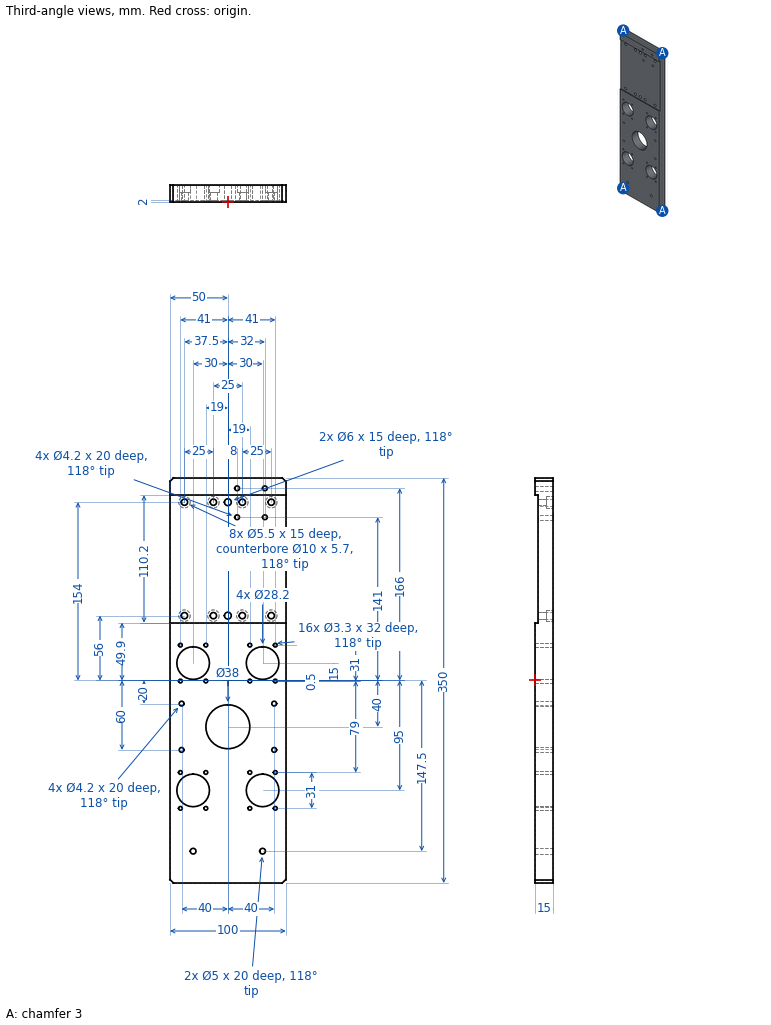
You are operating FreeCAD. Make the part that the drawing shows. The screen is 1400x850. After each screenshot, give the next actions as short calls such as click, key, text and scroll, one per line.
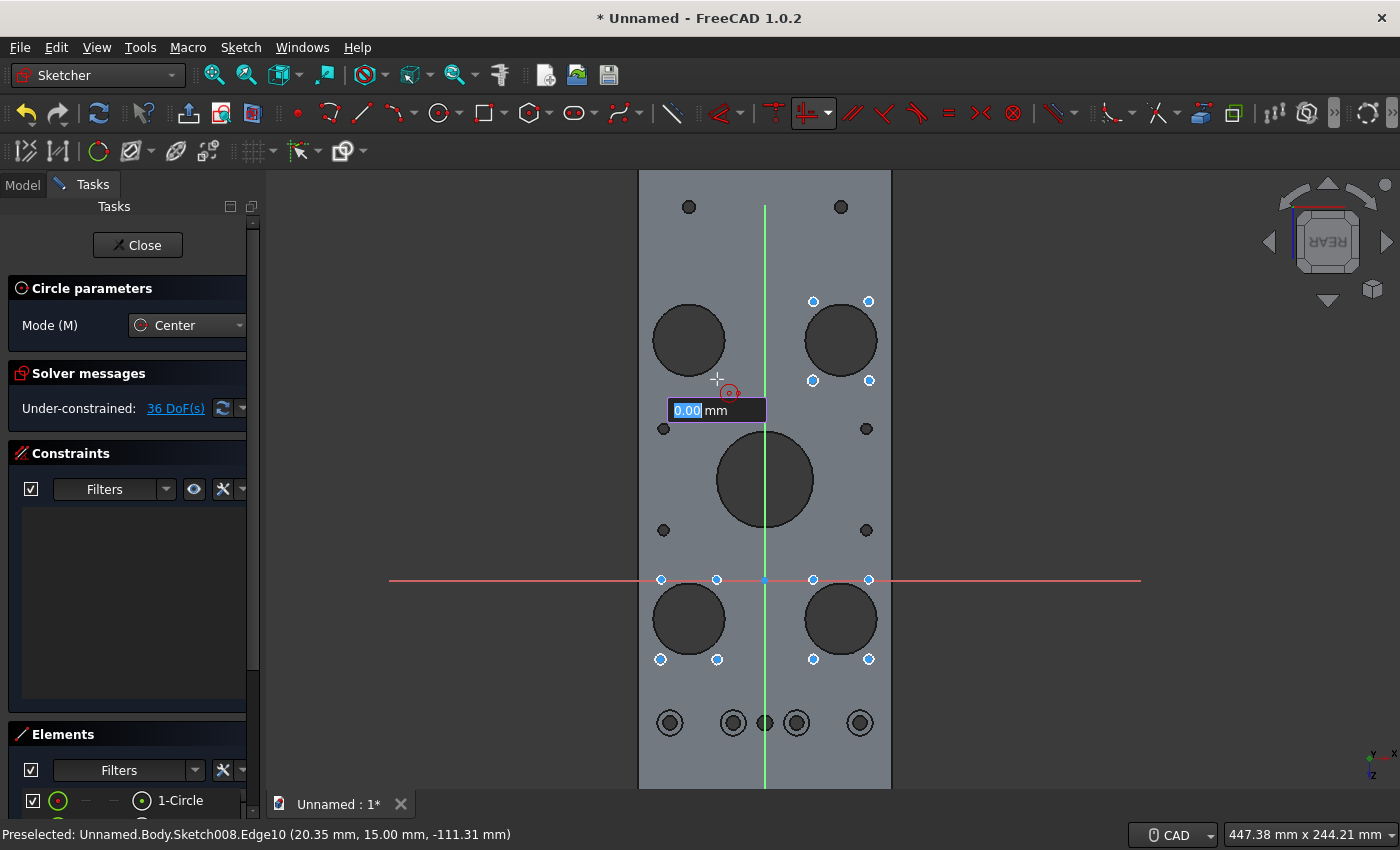
scroll(720, 377, up, 7)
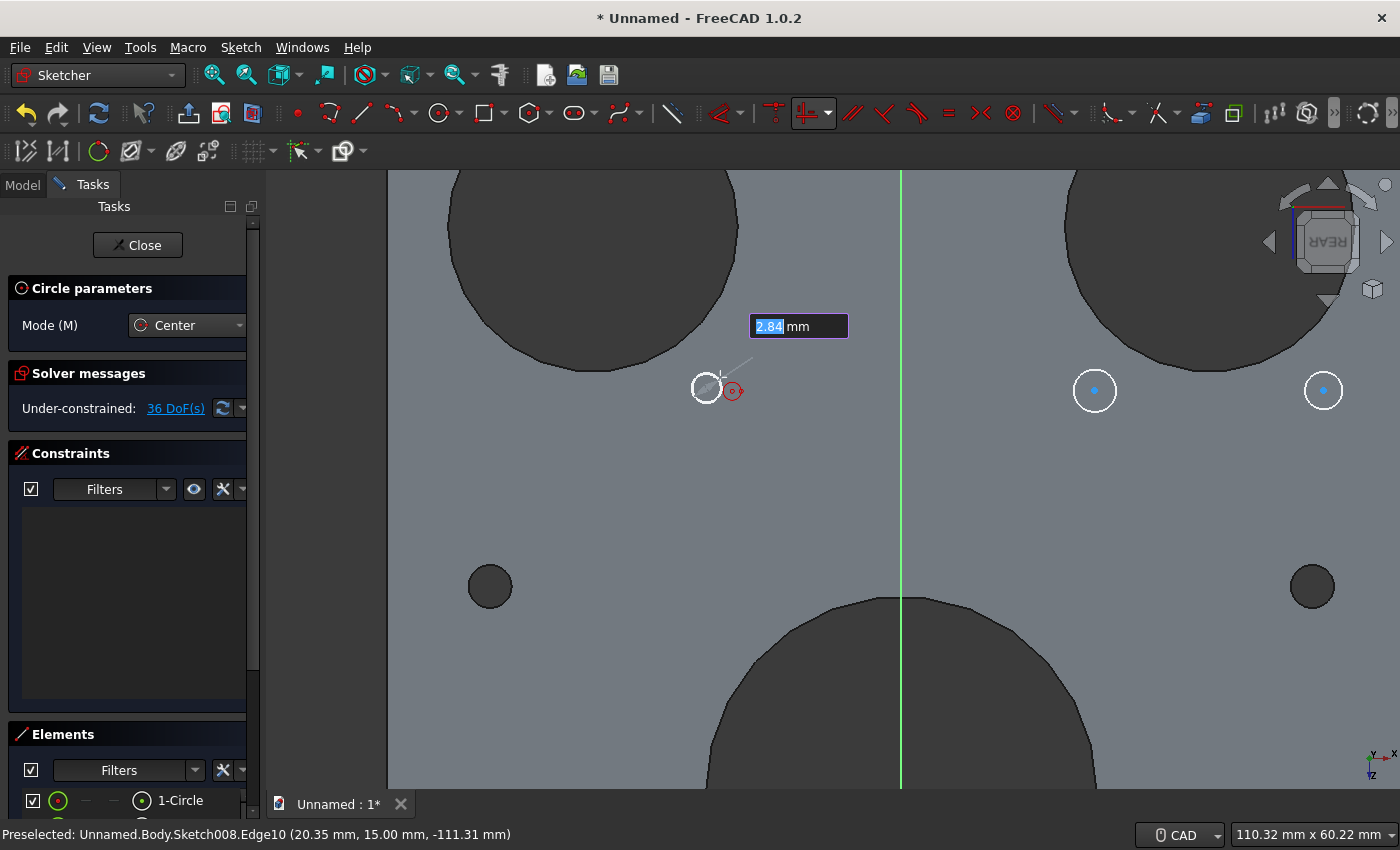
click(718, 374)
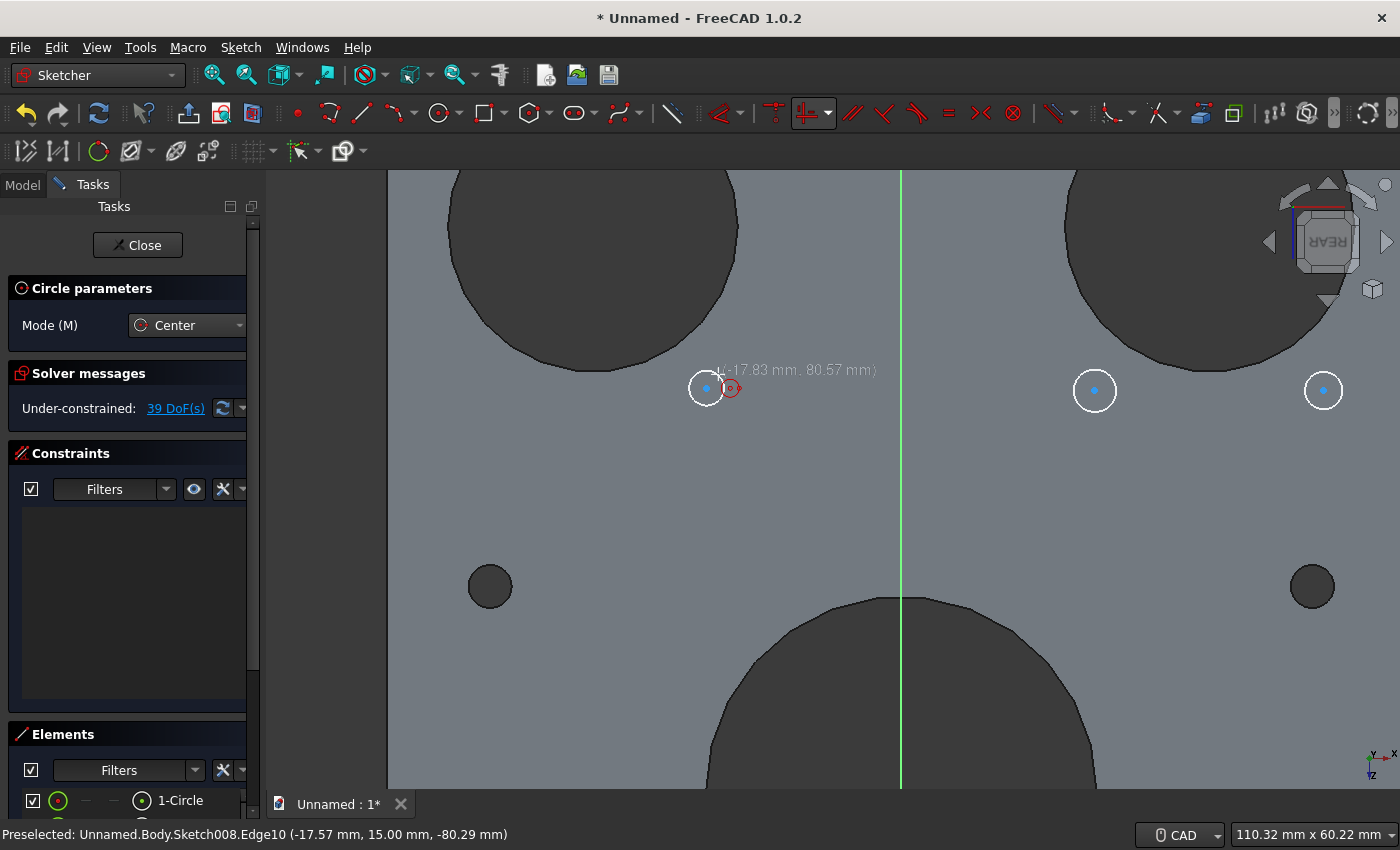
scroll(480, 386, up, 2)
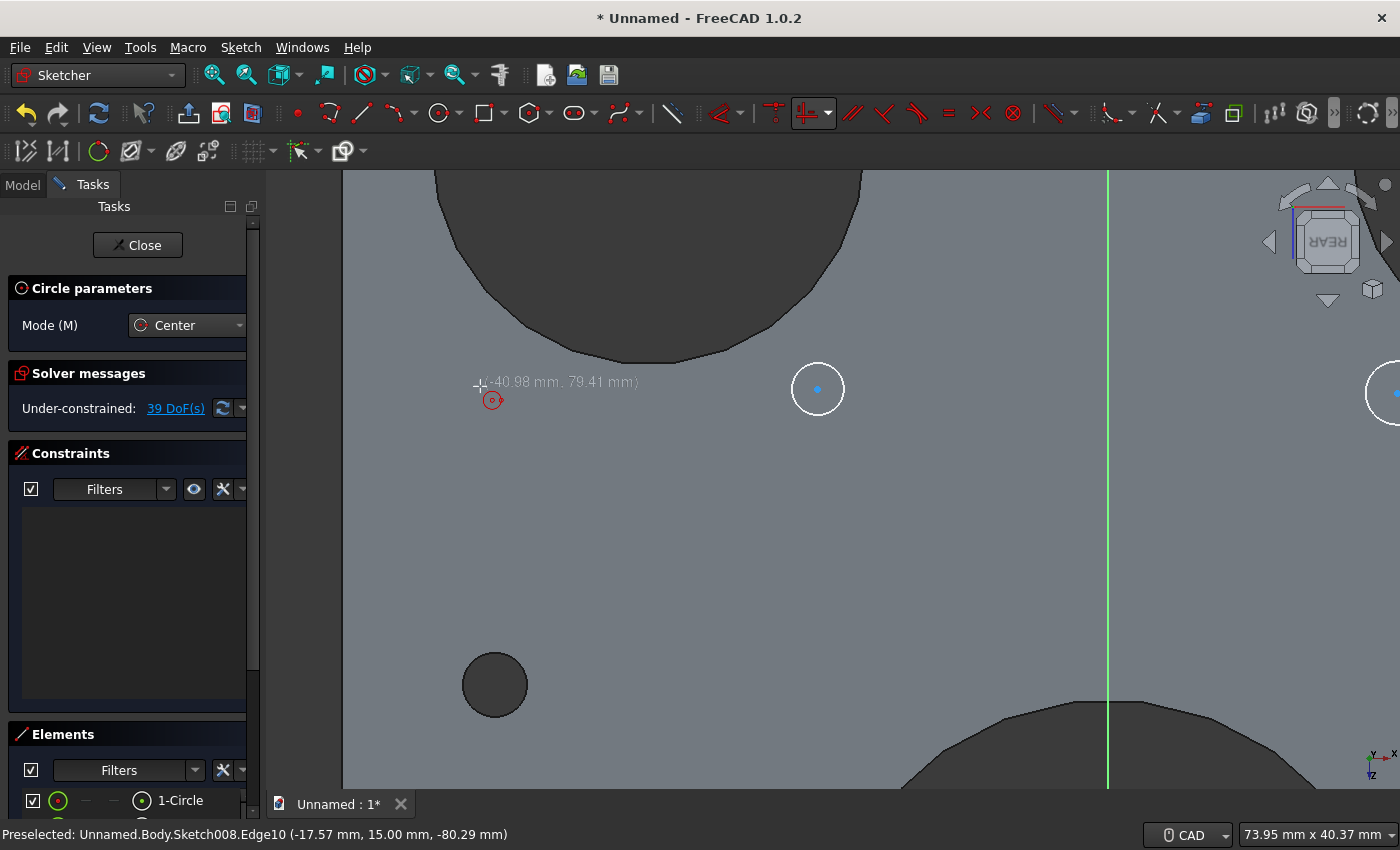
scroll(696, 378, down, 9)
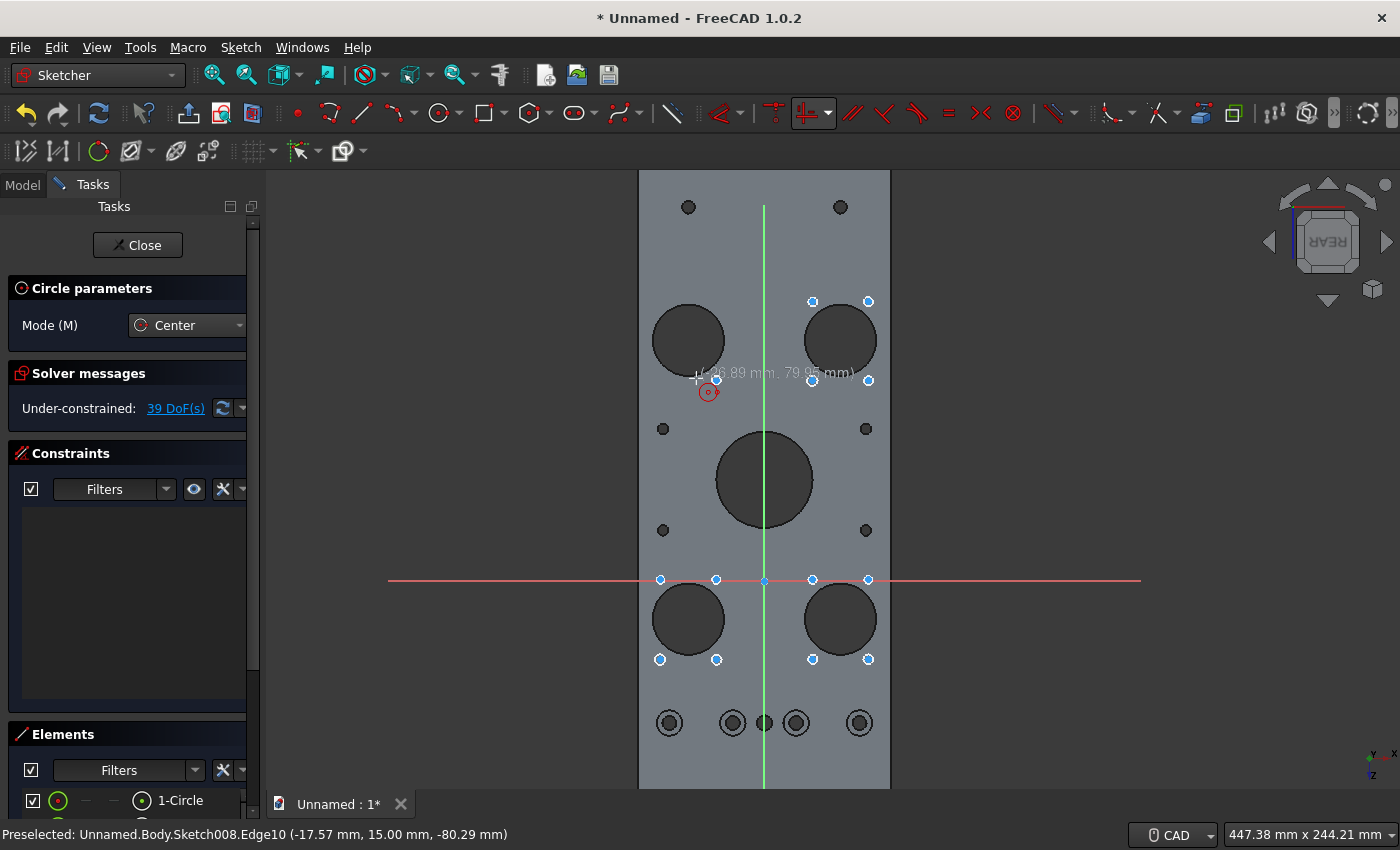
click(661, 380)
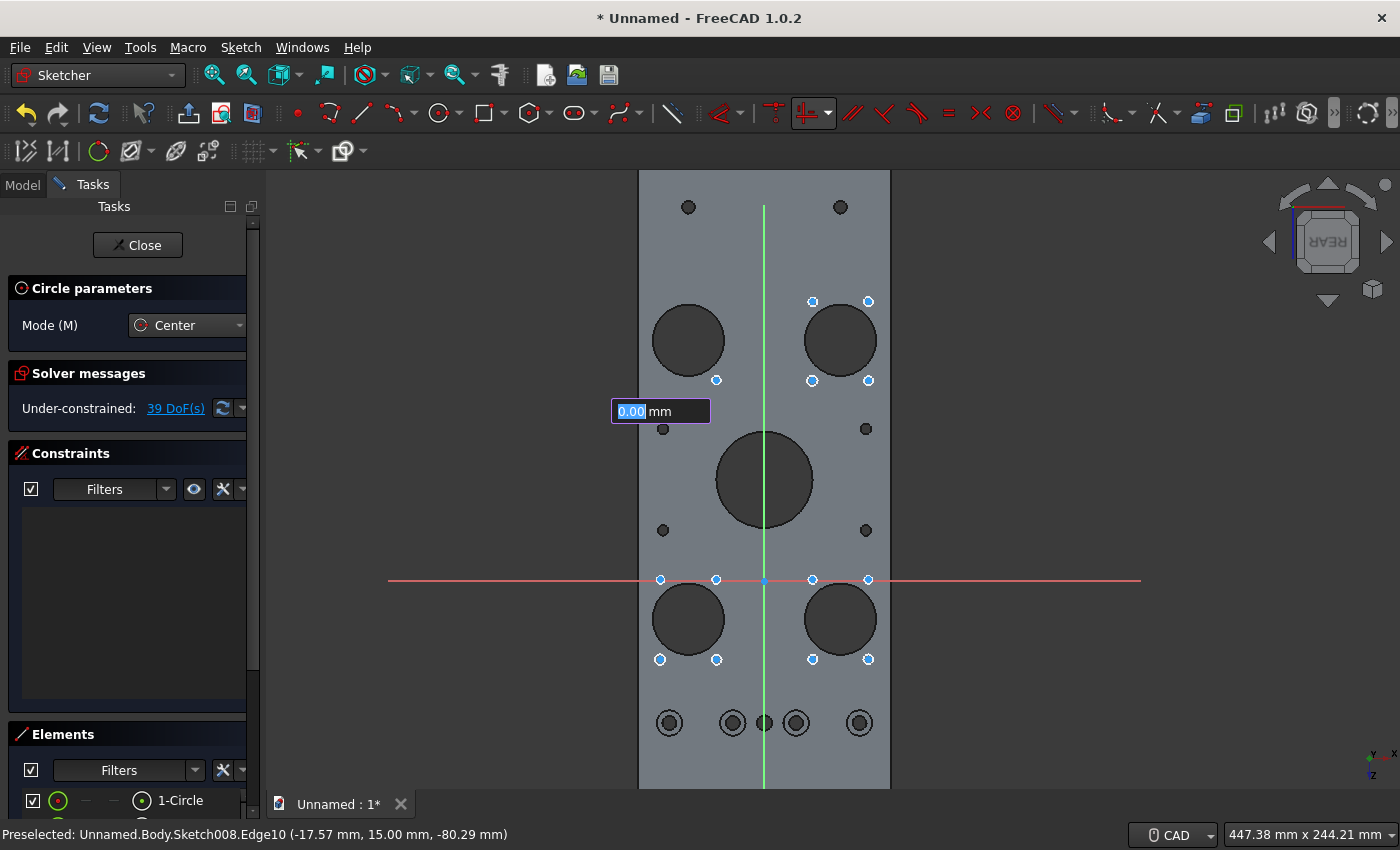
scroll(664, 377, up, 7)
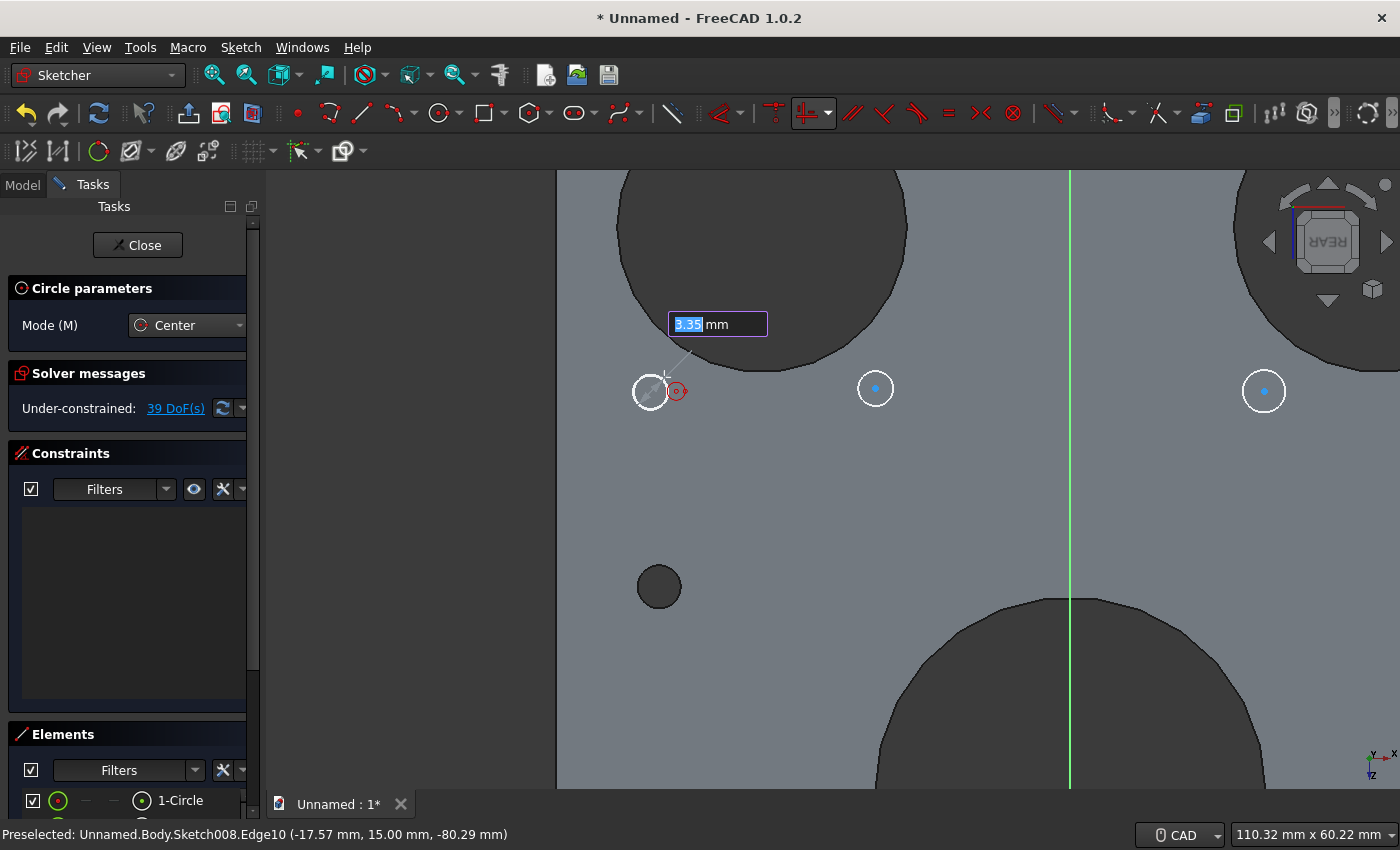
click(661, 374)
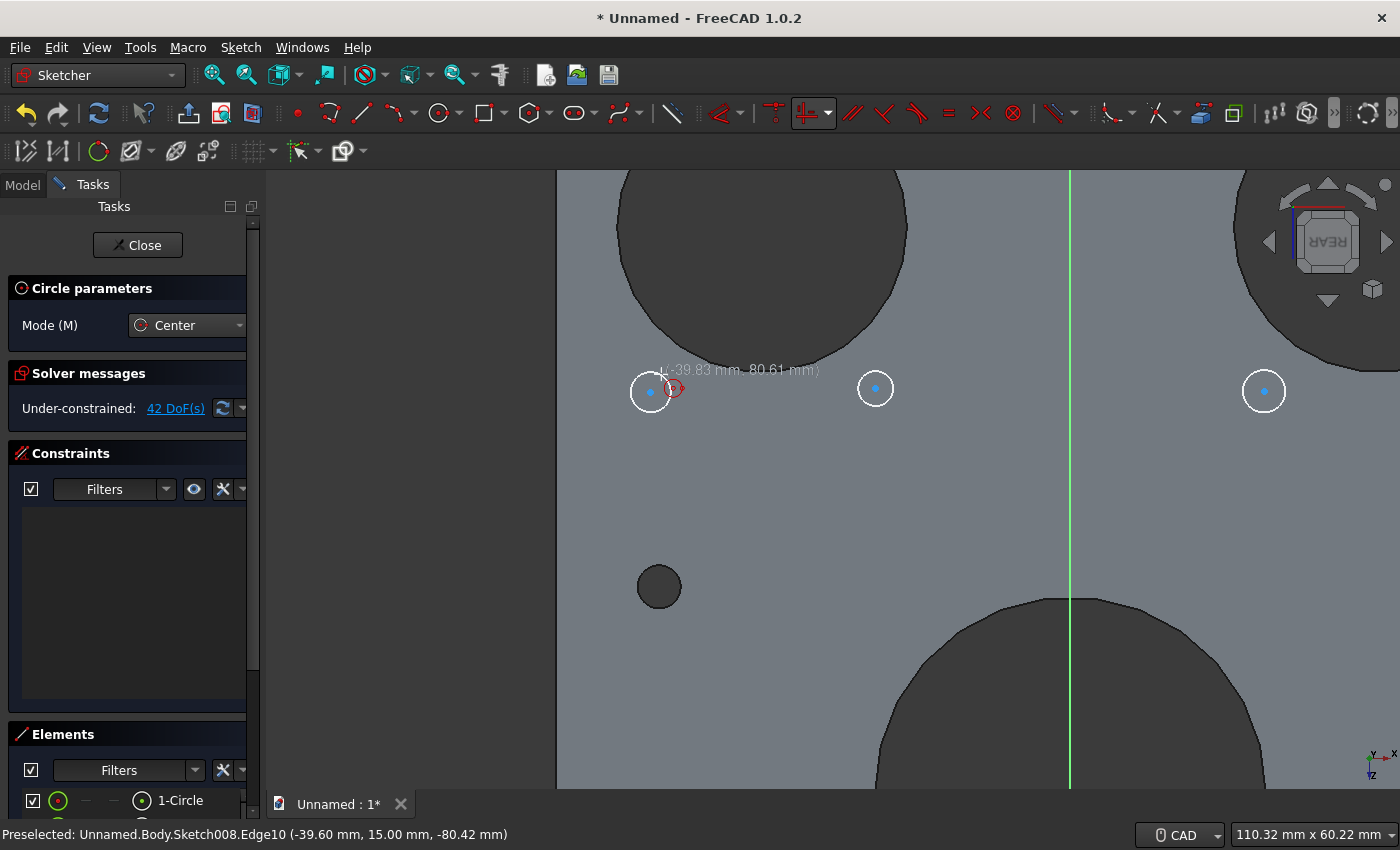
scroll(664, 377, down, 7)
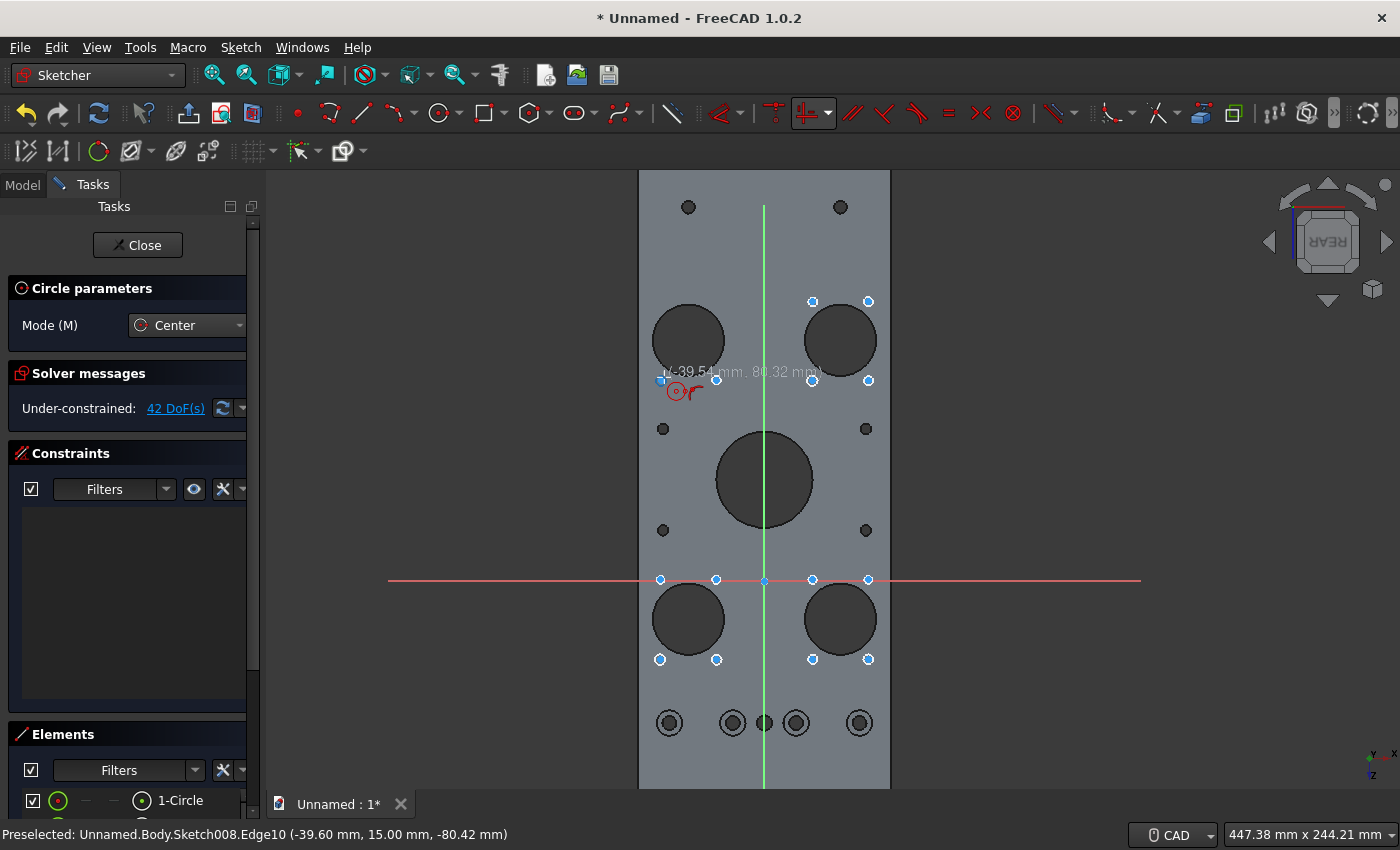
scroll(716, 301, up, 9)